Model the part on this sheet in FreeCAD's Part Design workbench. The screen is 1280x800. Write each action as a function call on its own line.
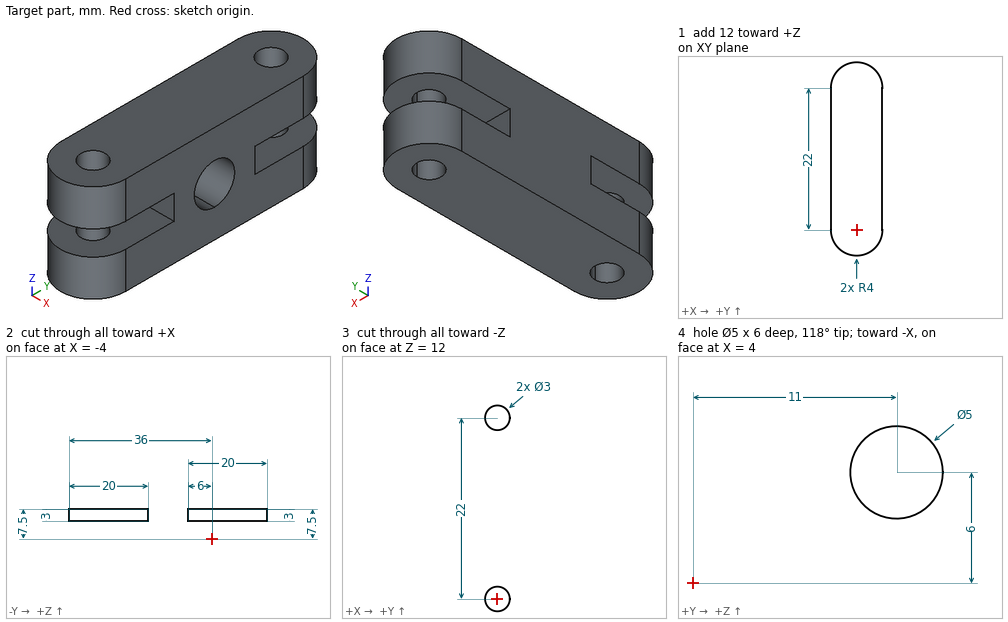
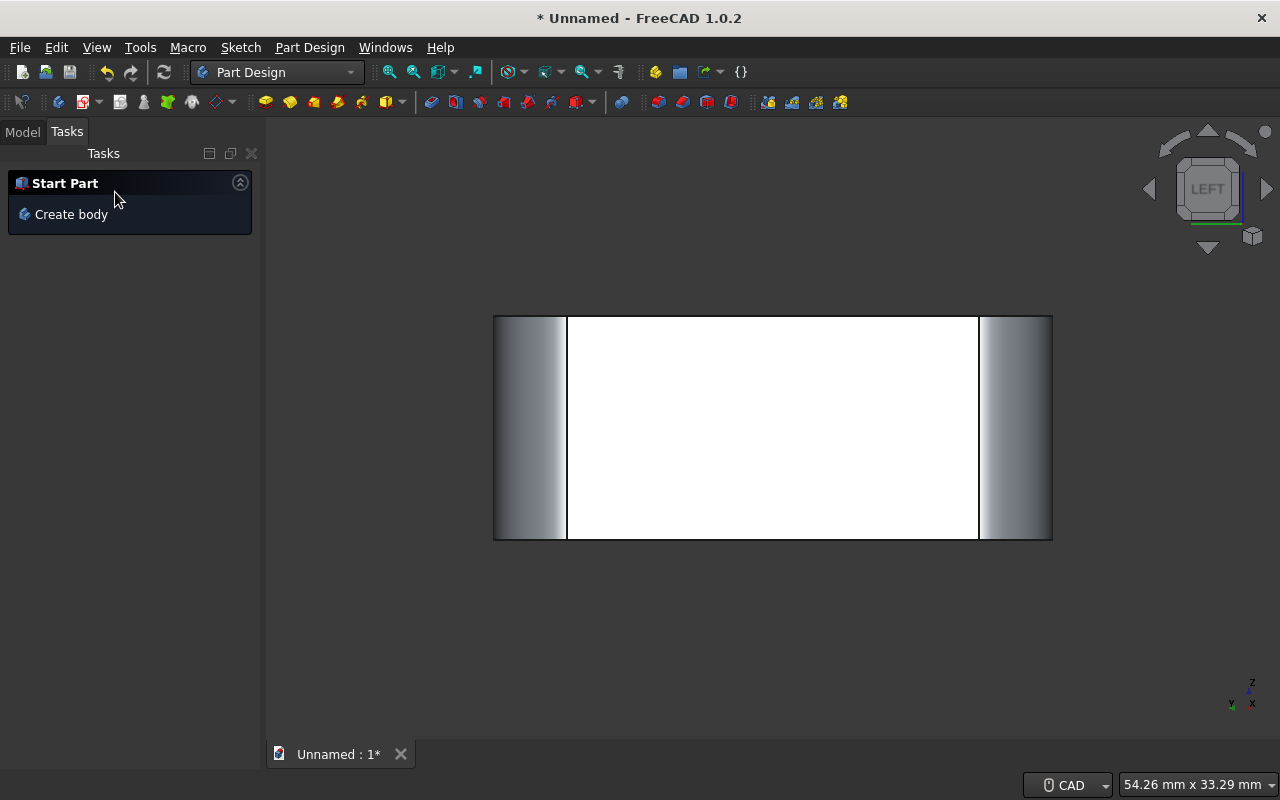
click(714, 427)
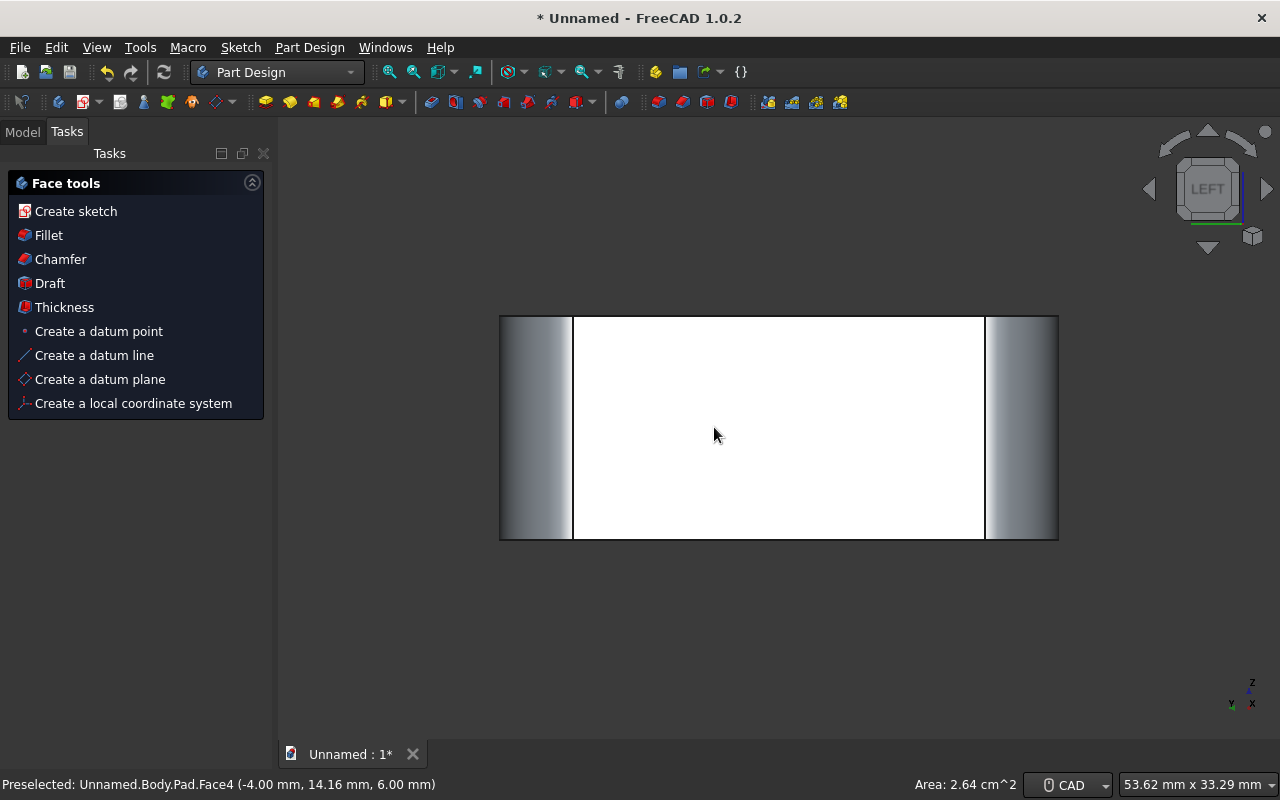
click(84, 102)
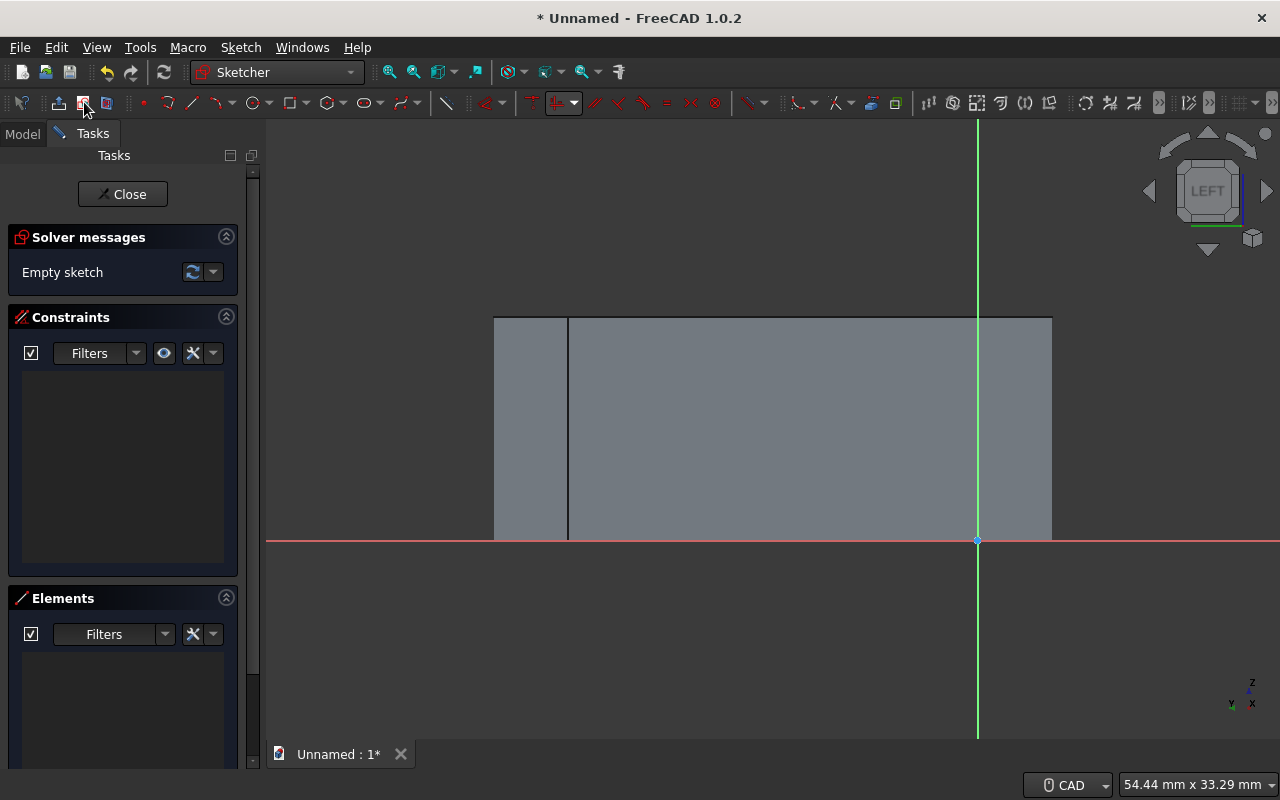
scroll(565, 344, down, 2)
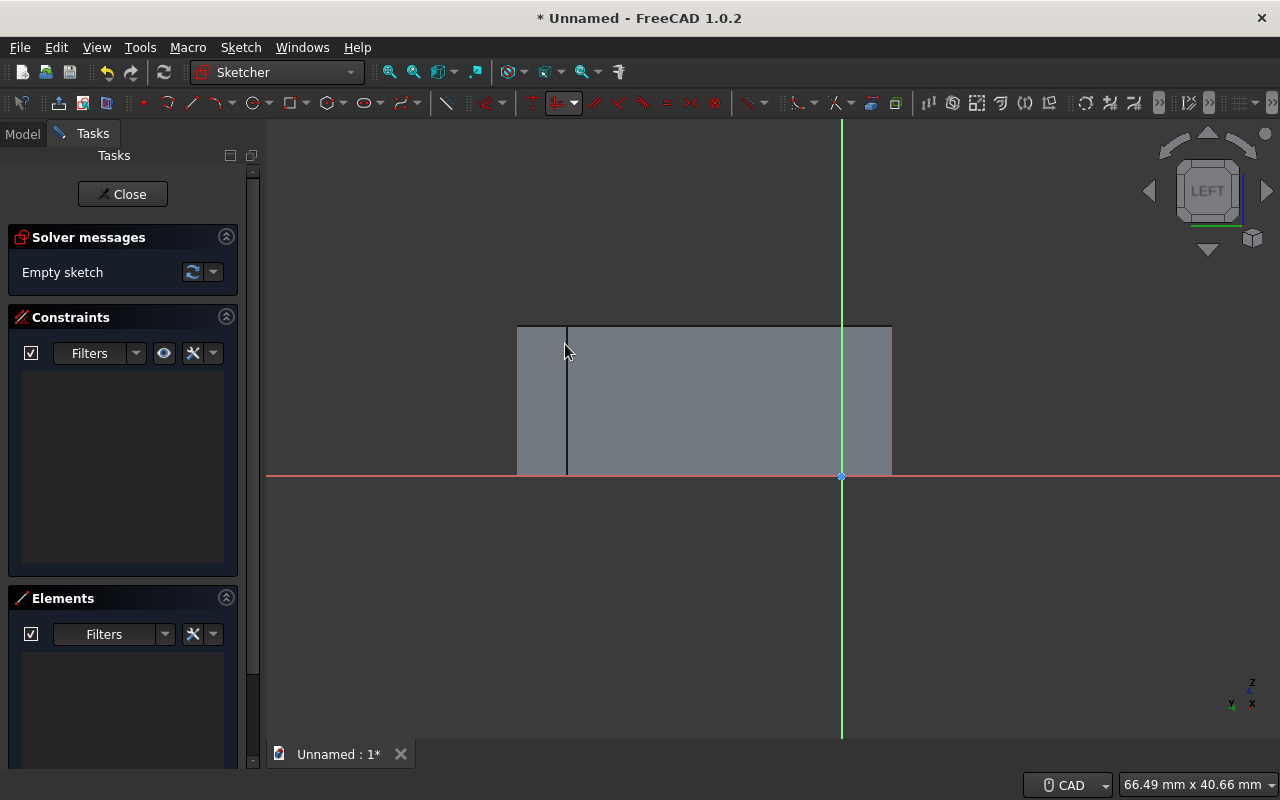
key(g)
key(r)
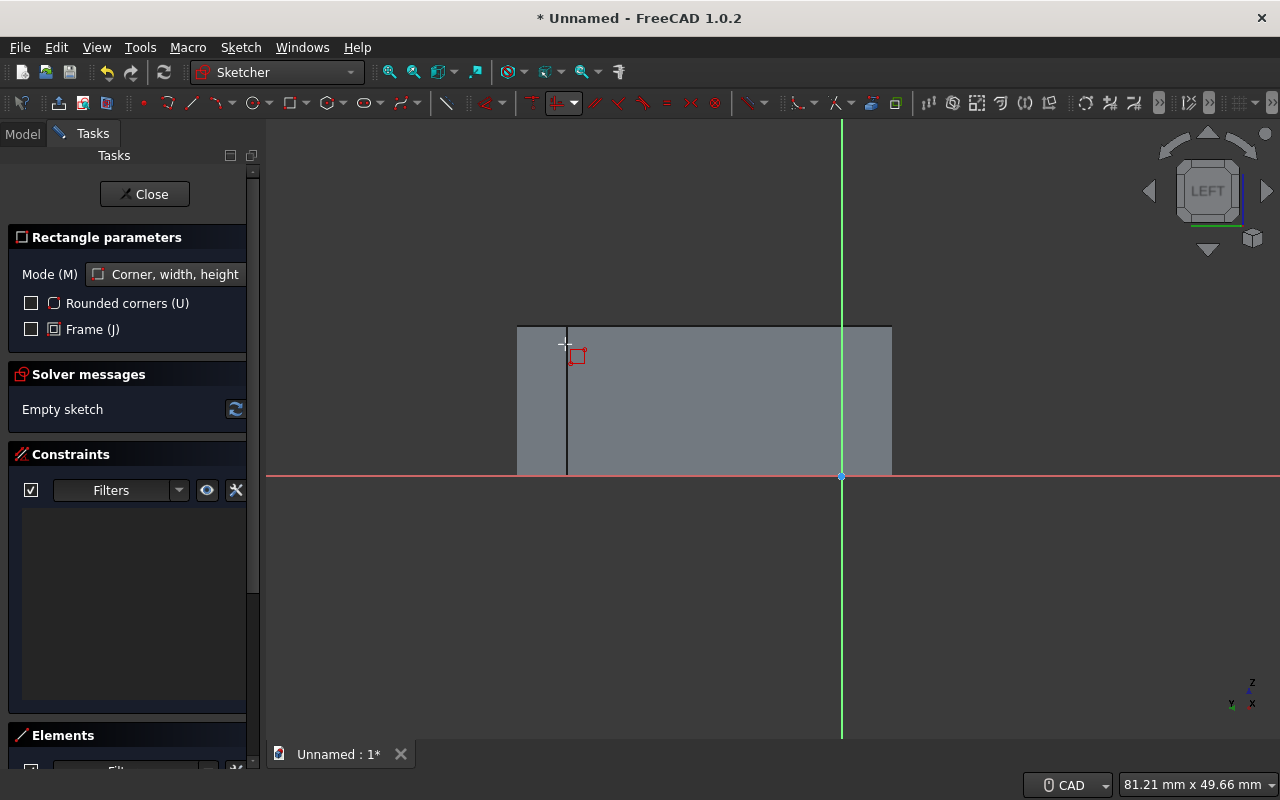
click(392, 382)
move(642, 420)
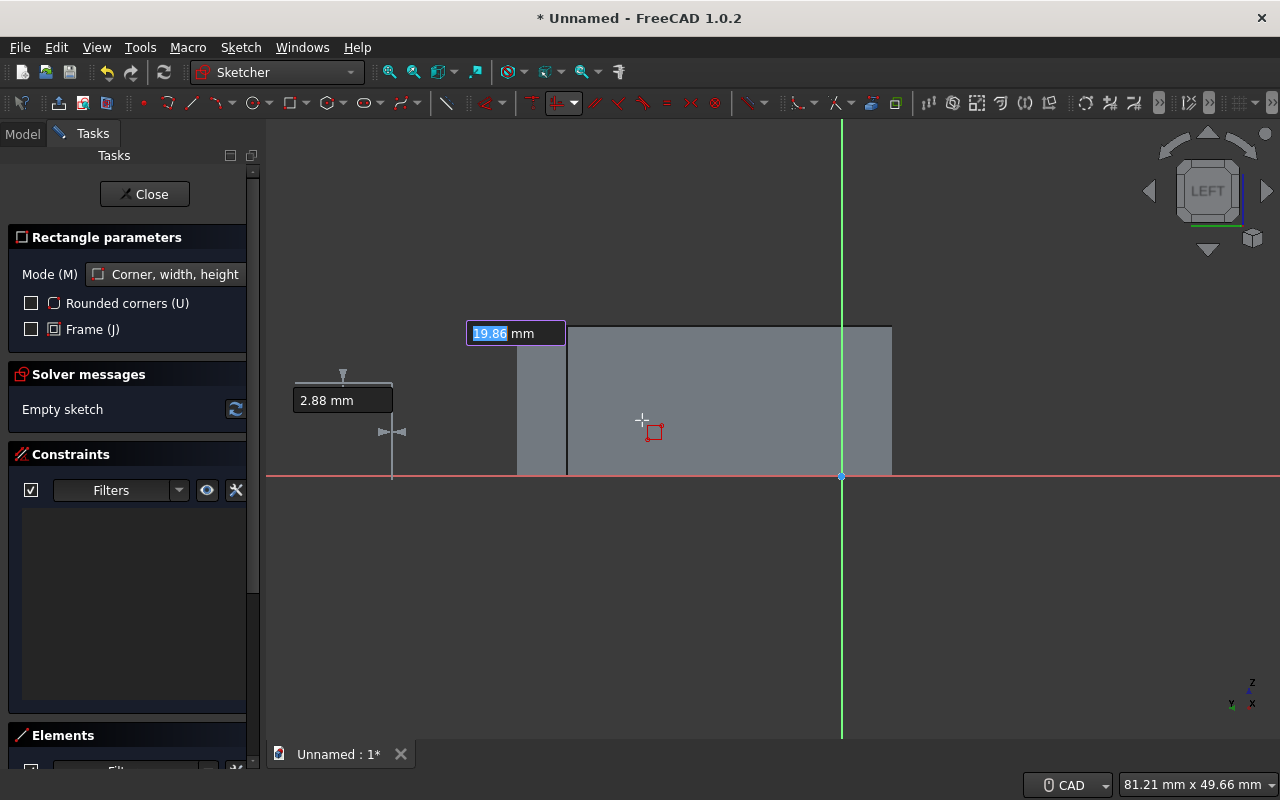
text(20)
key(Tab)
text(3)
key(Return)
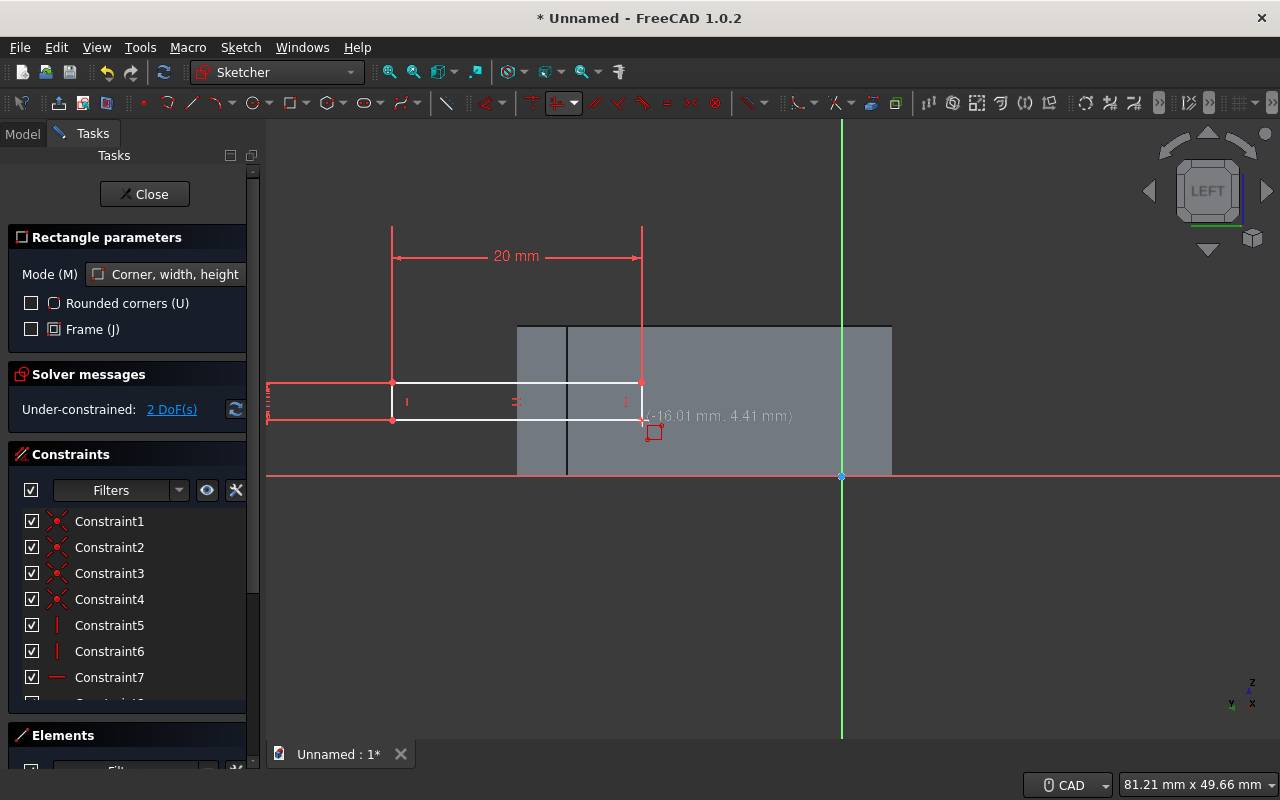
click(767, 382)
move(1017, 420)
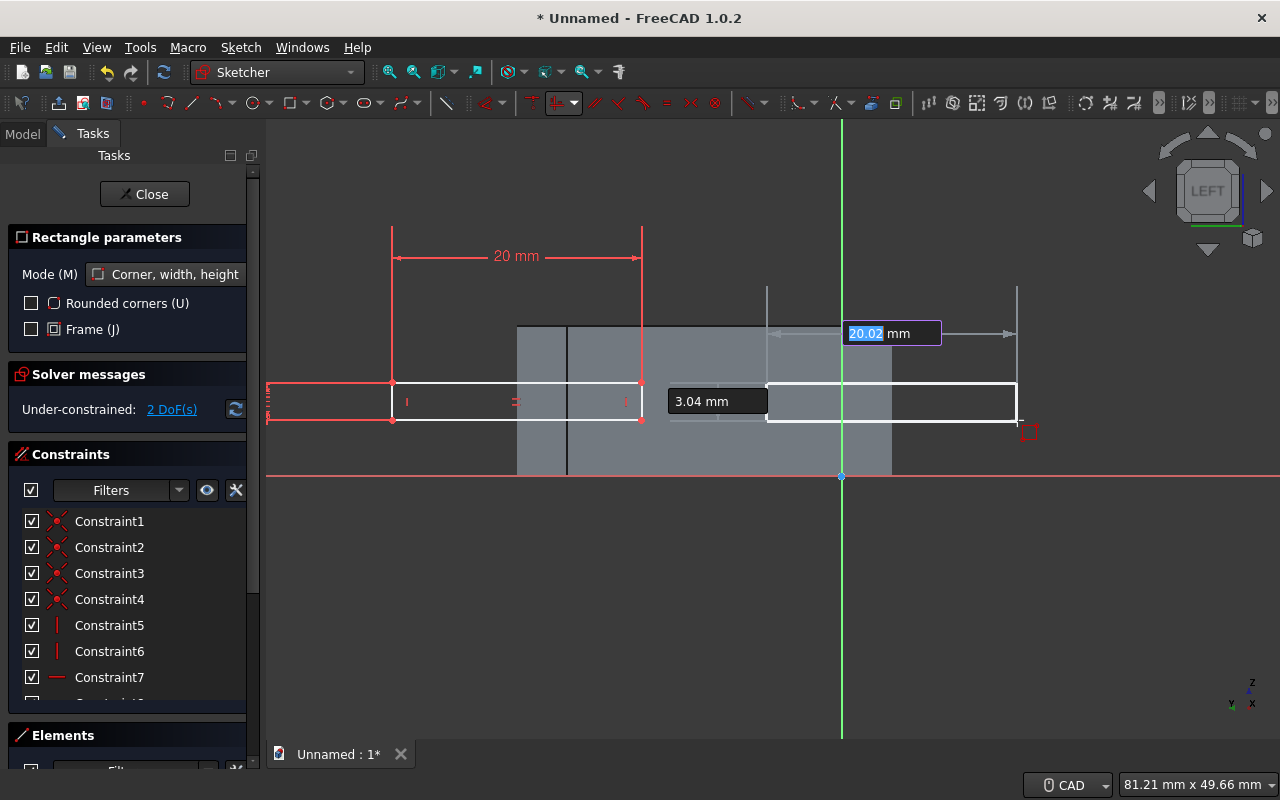
text(20)
key(Tab)
text(3)
key(Return)
key(Escape)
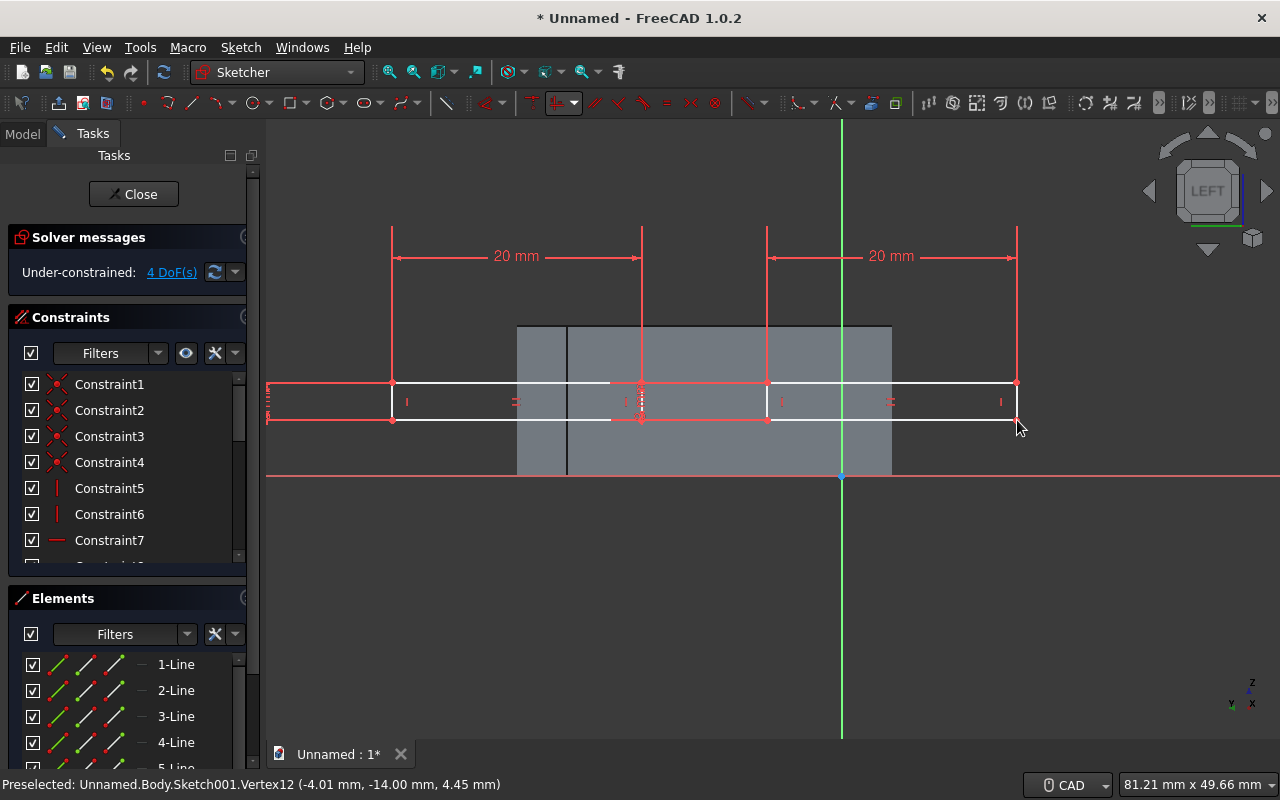
click(486, 104)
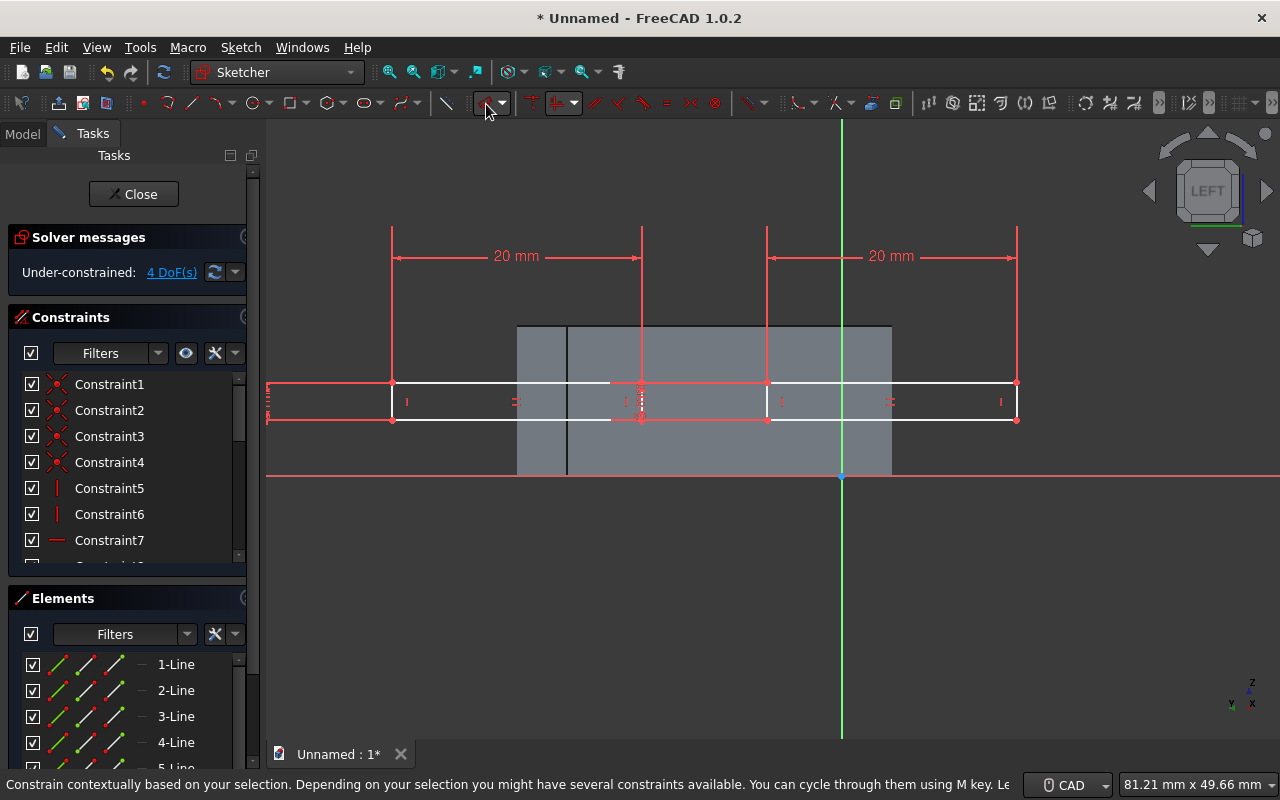
click(767, 383)
click(804, 510)